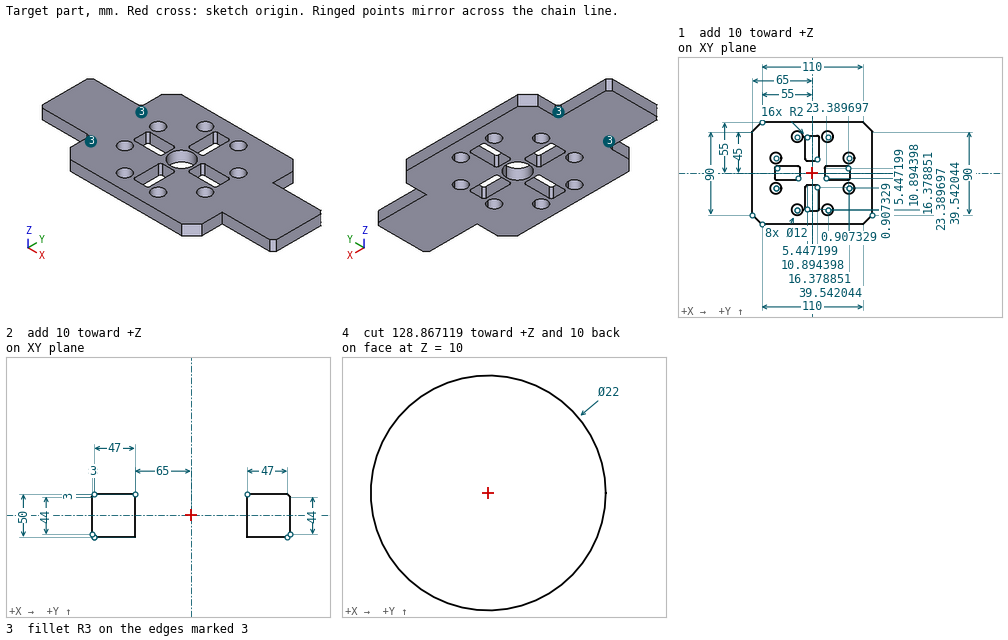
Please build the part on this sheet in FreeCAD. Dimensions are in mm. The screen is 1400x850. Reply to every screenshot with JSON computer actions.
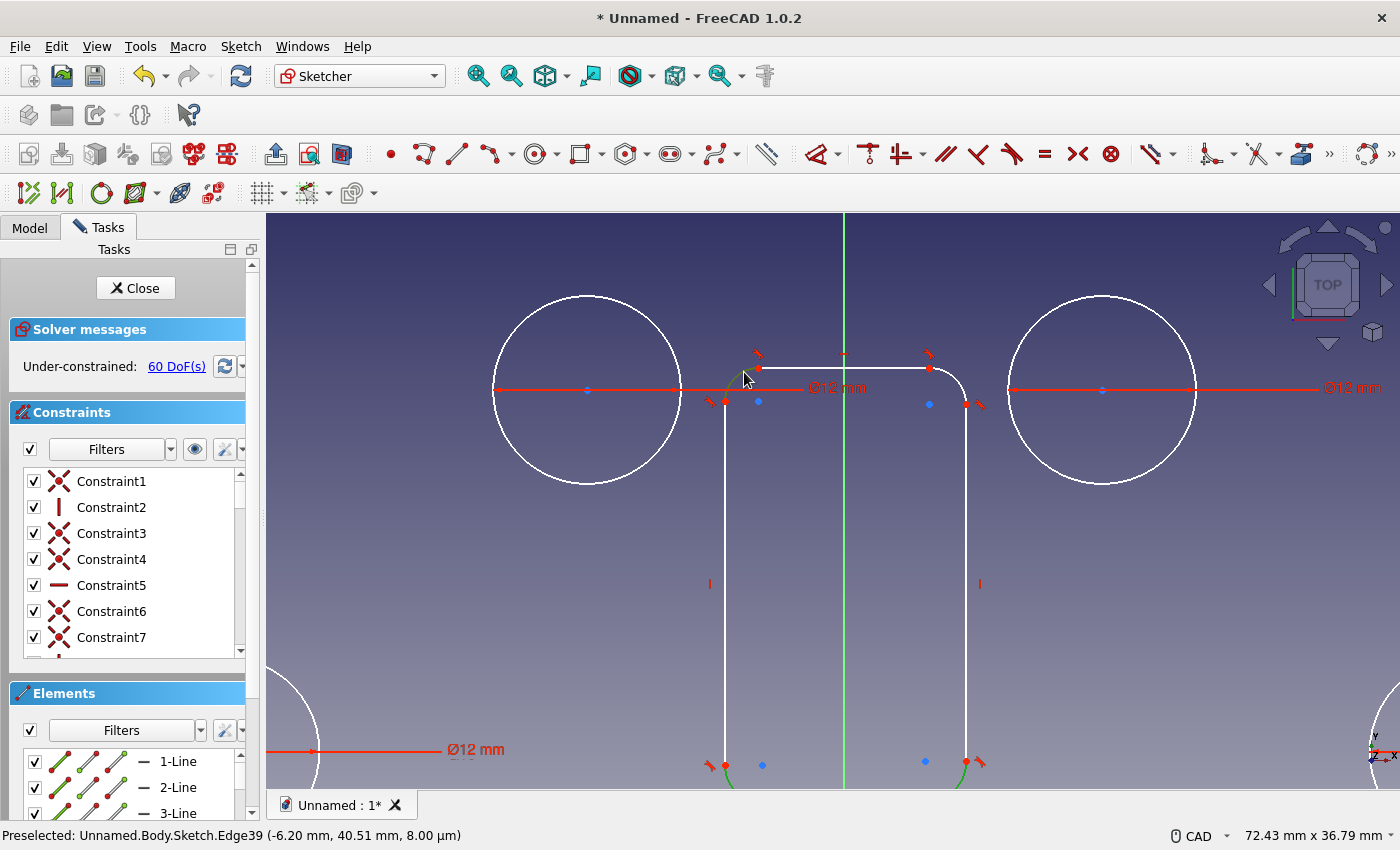
{"action": "left_click", "coordinate": [962, 388]}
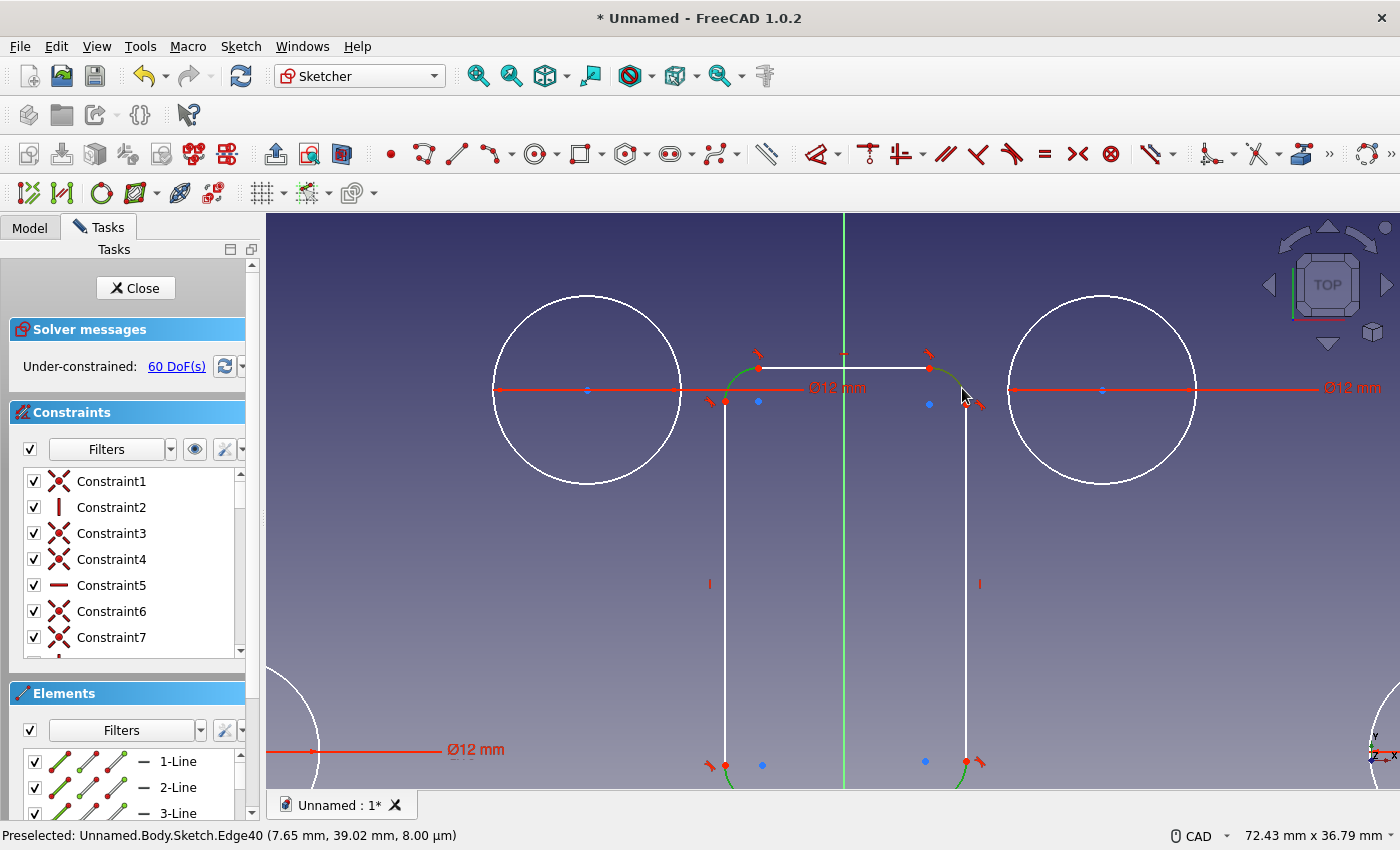
{"action": "left_click", "coordinate": [1045, 154]}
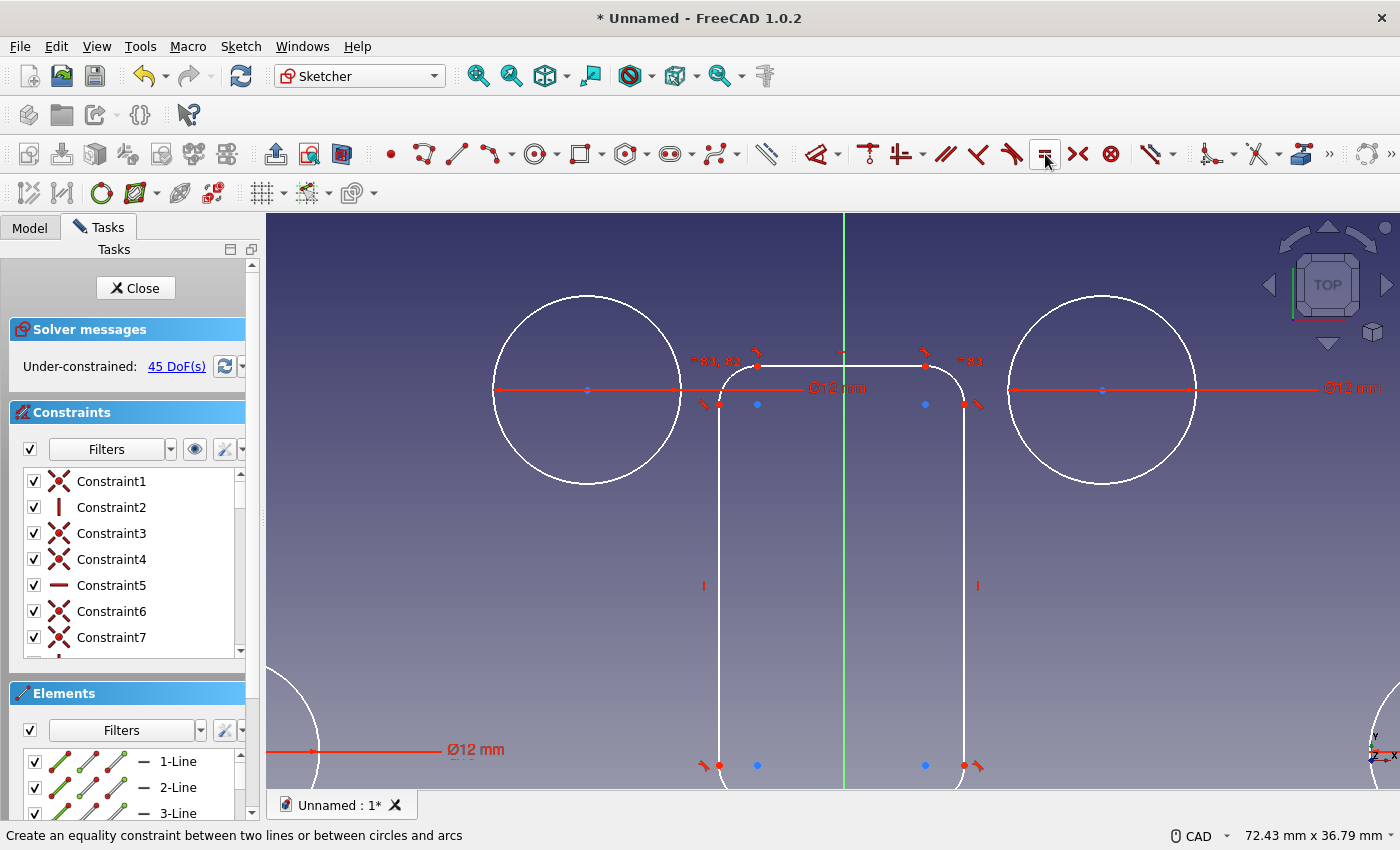
{"action": "scroll", "coordinate": [744, 374], "scroll_direction": "down", "scroll_amount": 8}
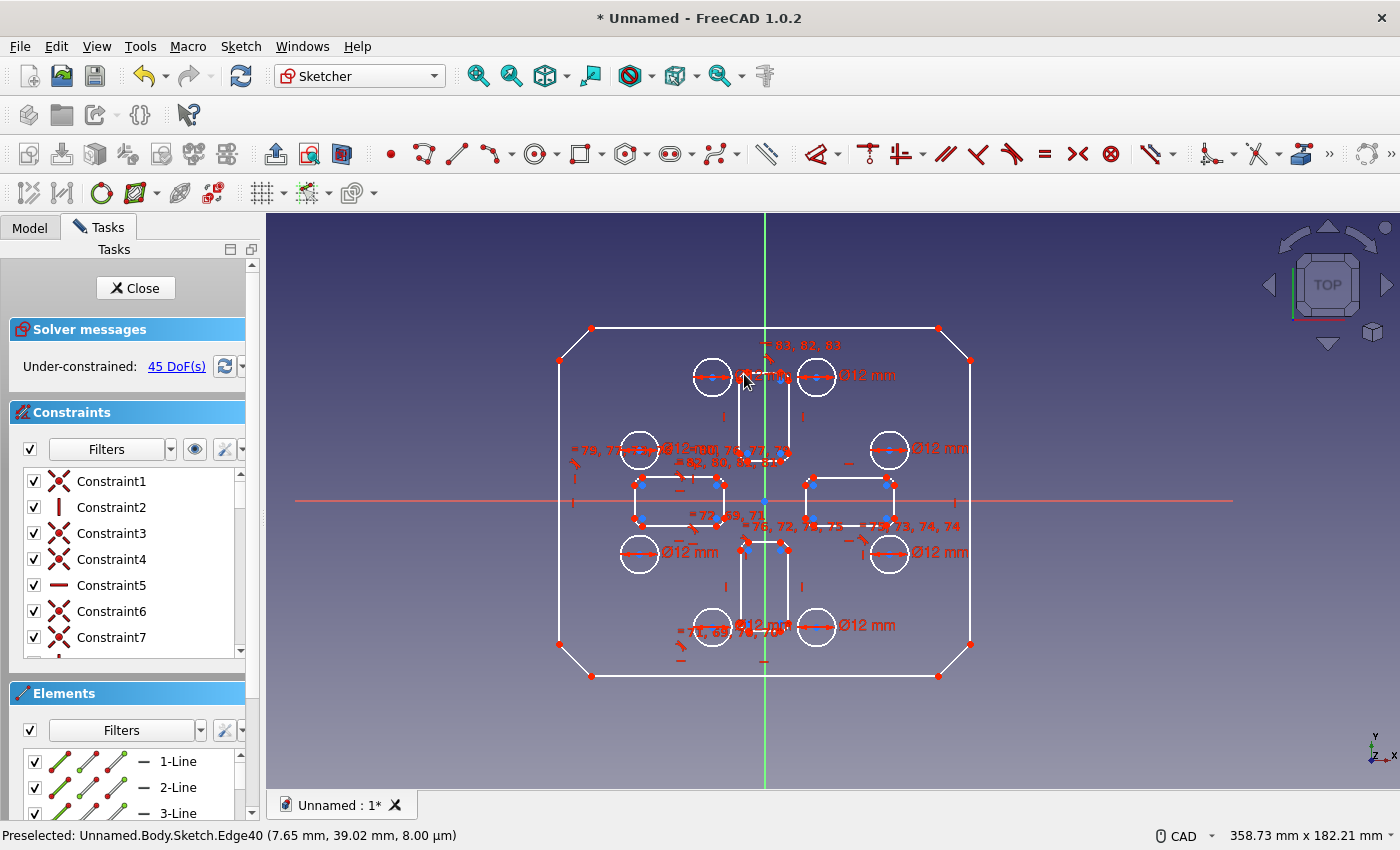
{"action": "scroll", "coordinate": [814, 518], "scroll_direction": "up", "scroll_amount": 3}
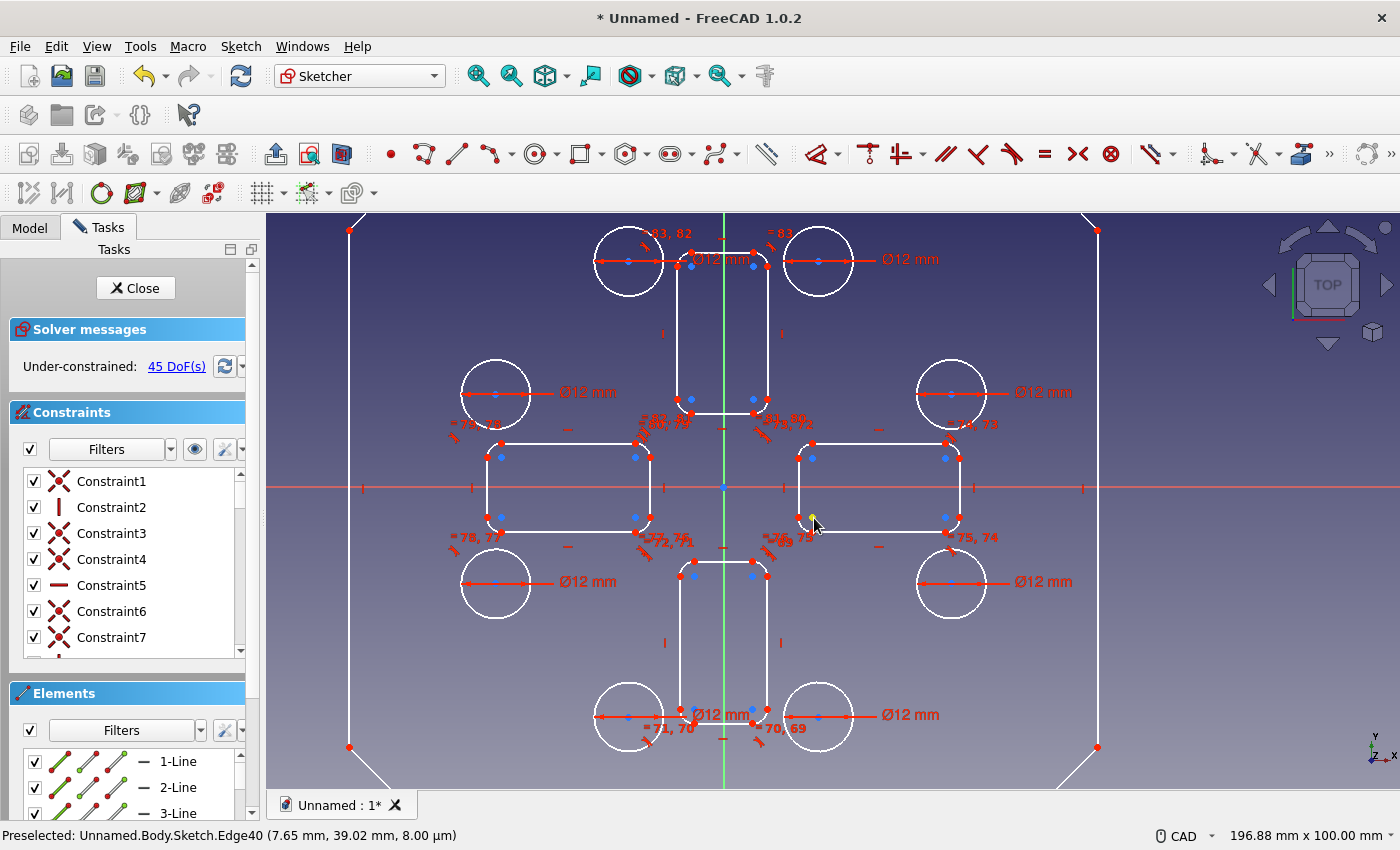
{"action": "left_click", "coordinate": [813, 518]}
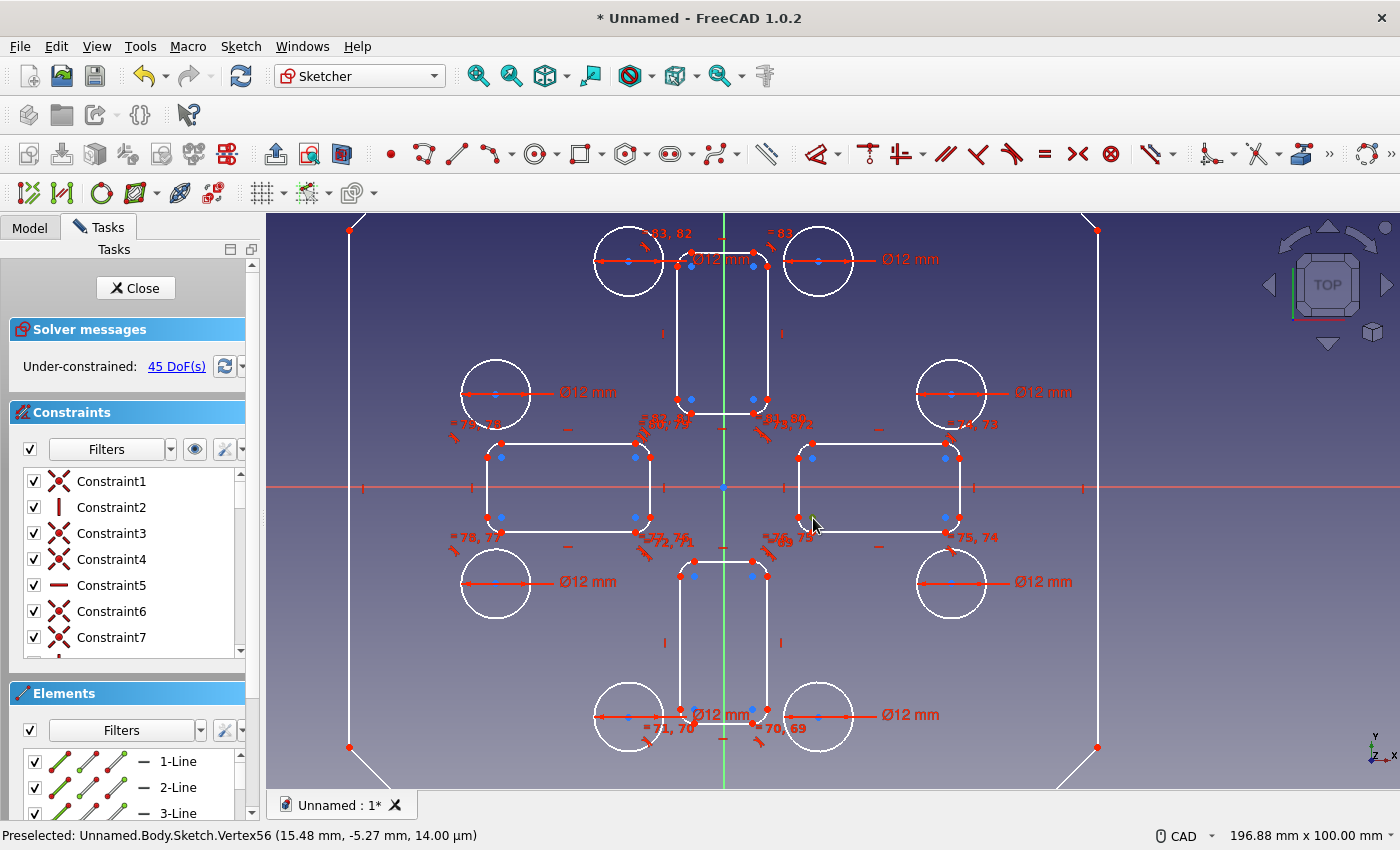
{"action": "left_click", "coordinate": [636, 518]}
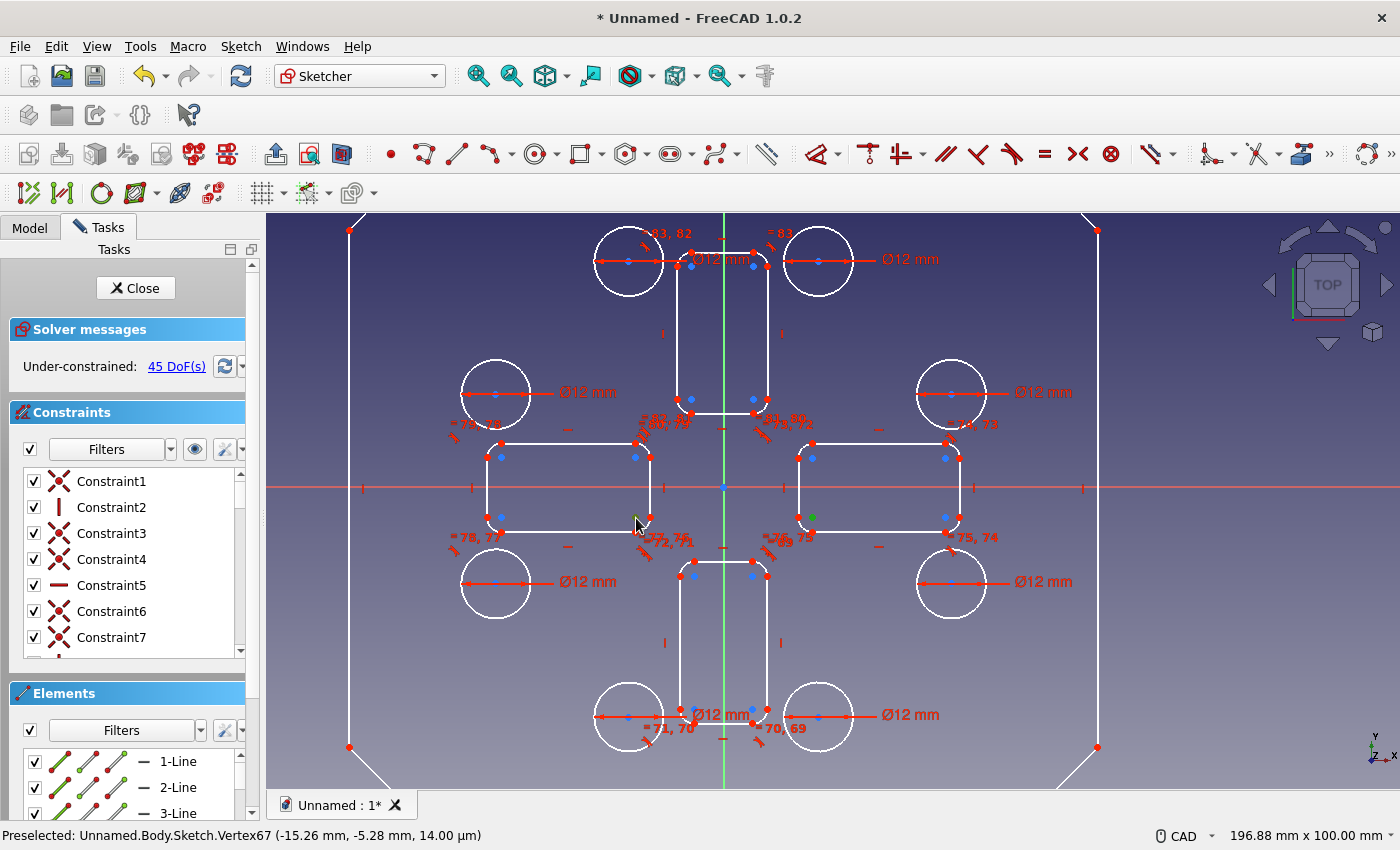
{"action": "left_click", "coordinate": [724, 687]}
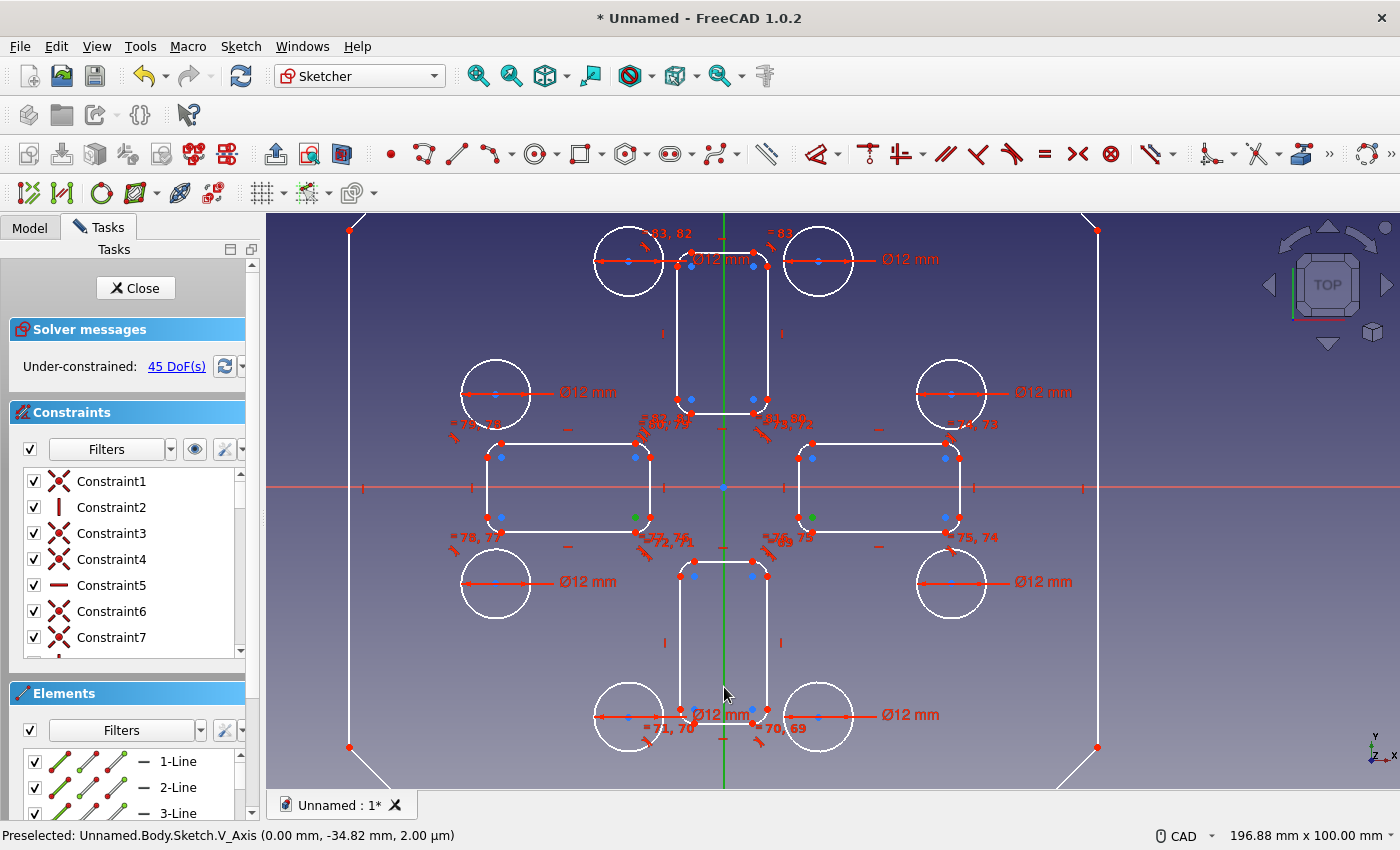
{"action": "left_click", "coordinate": [1078, 154]}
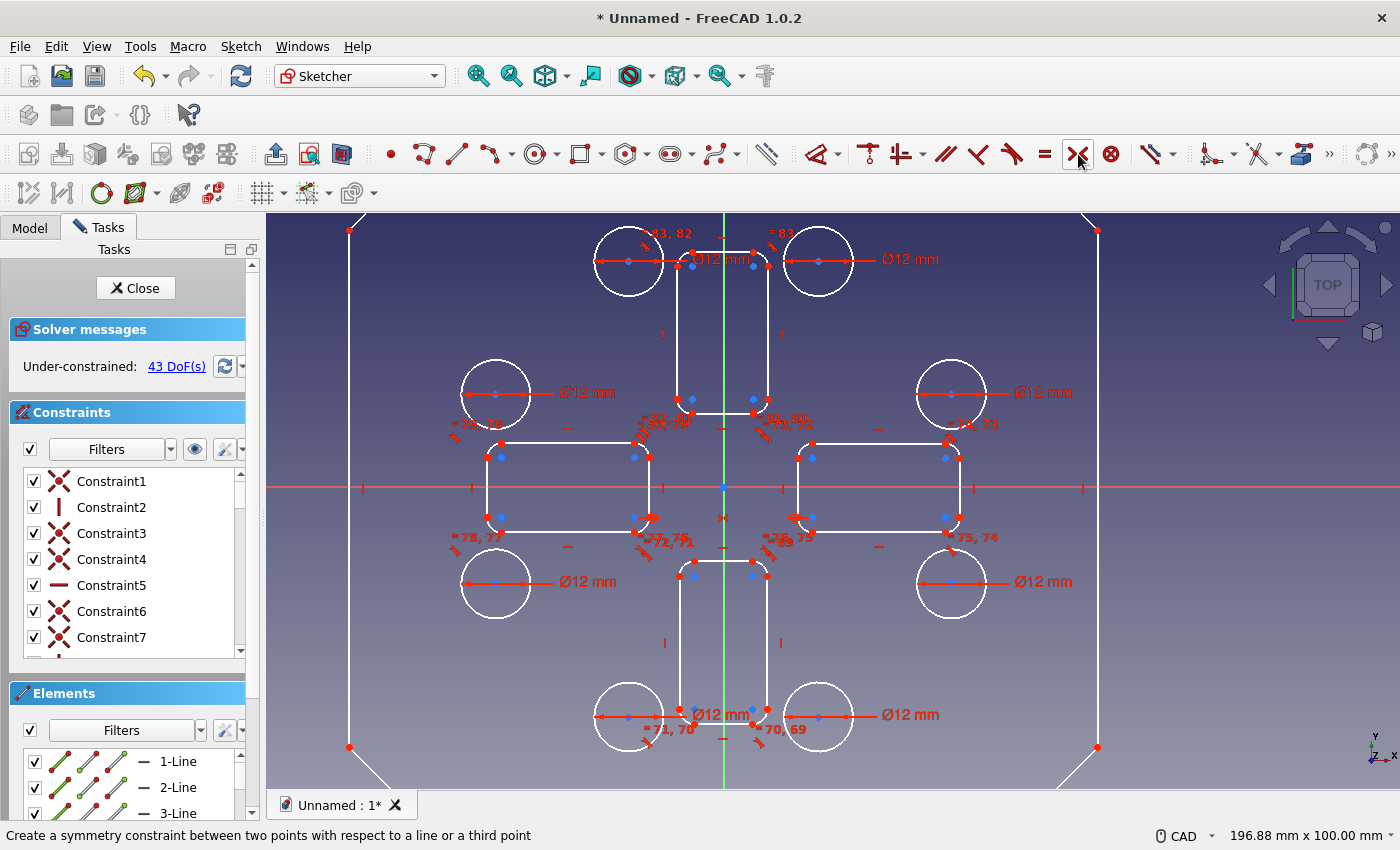
{"action": "left_click", "coordinate": [945, 458]}